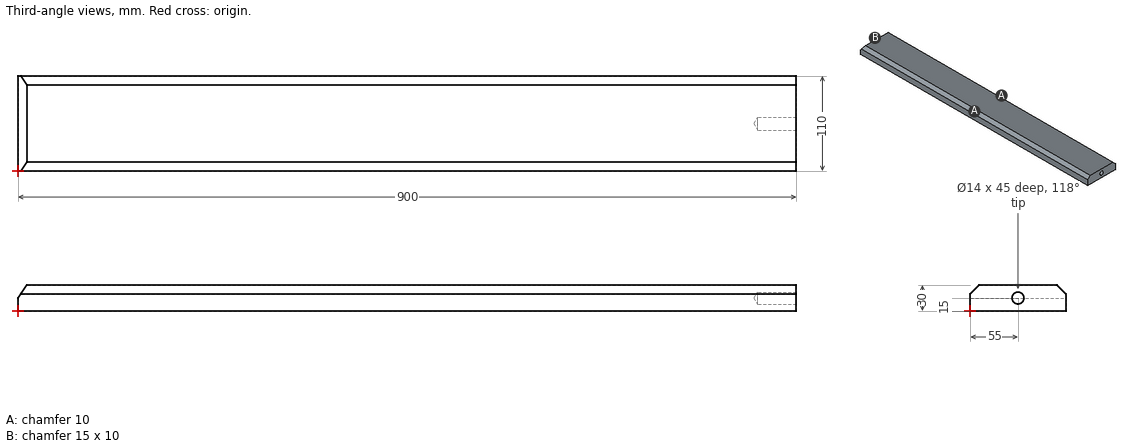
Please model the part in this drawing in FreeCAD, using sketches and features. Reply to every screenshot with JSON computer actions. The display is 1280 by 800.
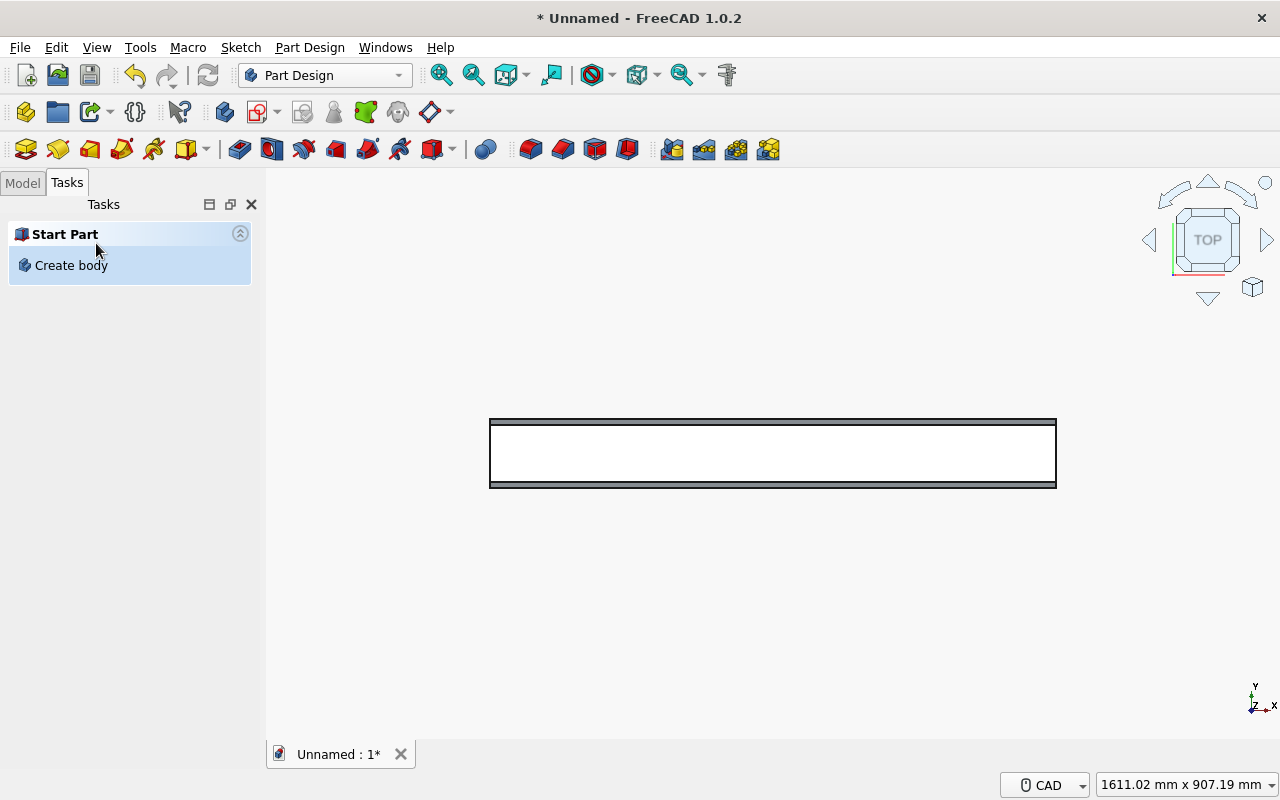
{"action": "left_click", "coordinate": [490, 452]}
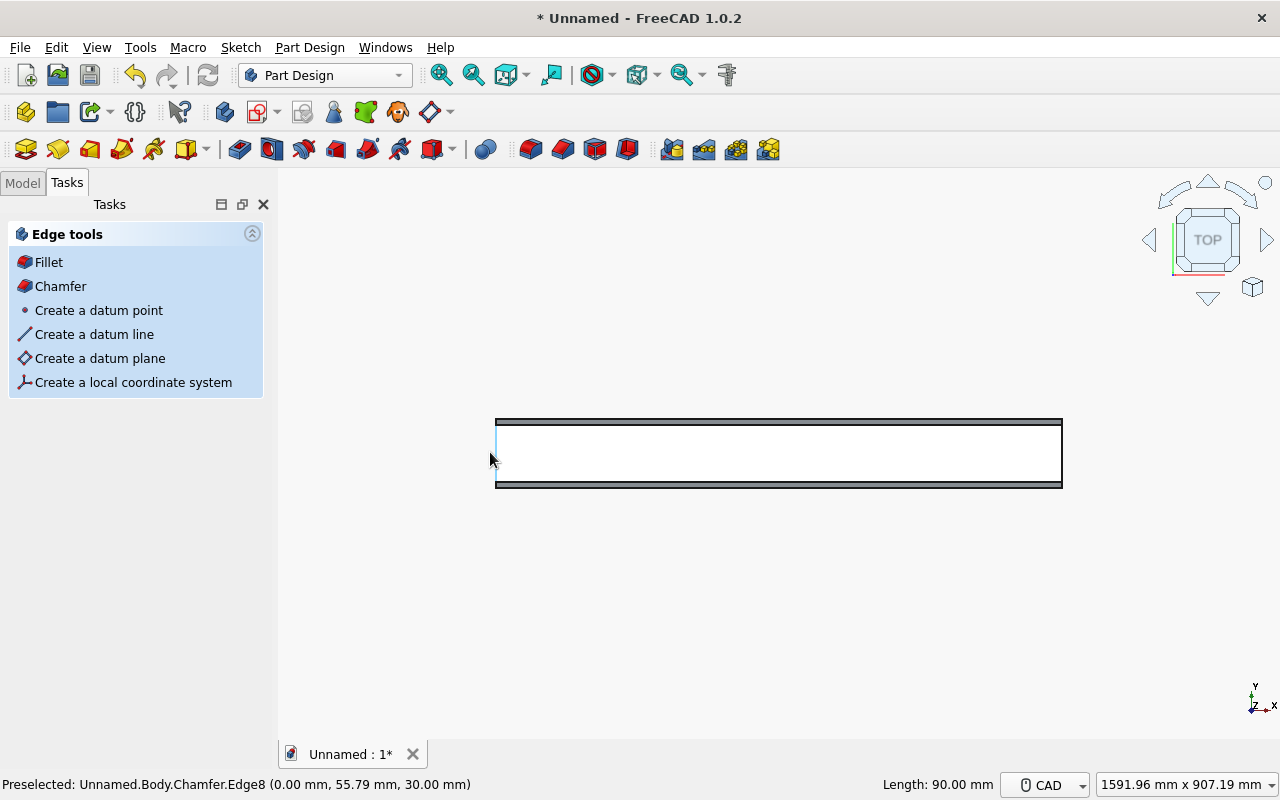
{"action": "left_click", "coordinate": [564, 150]}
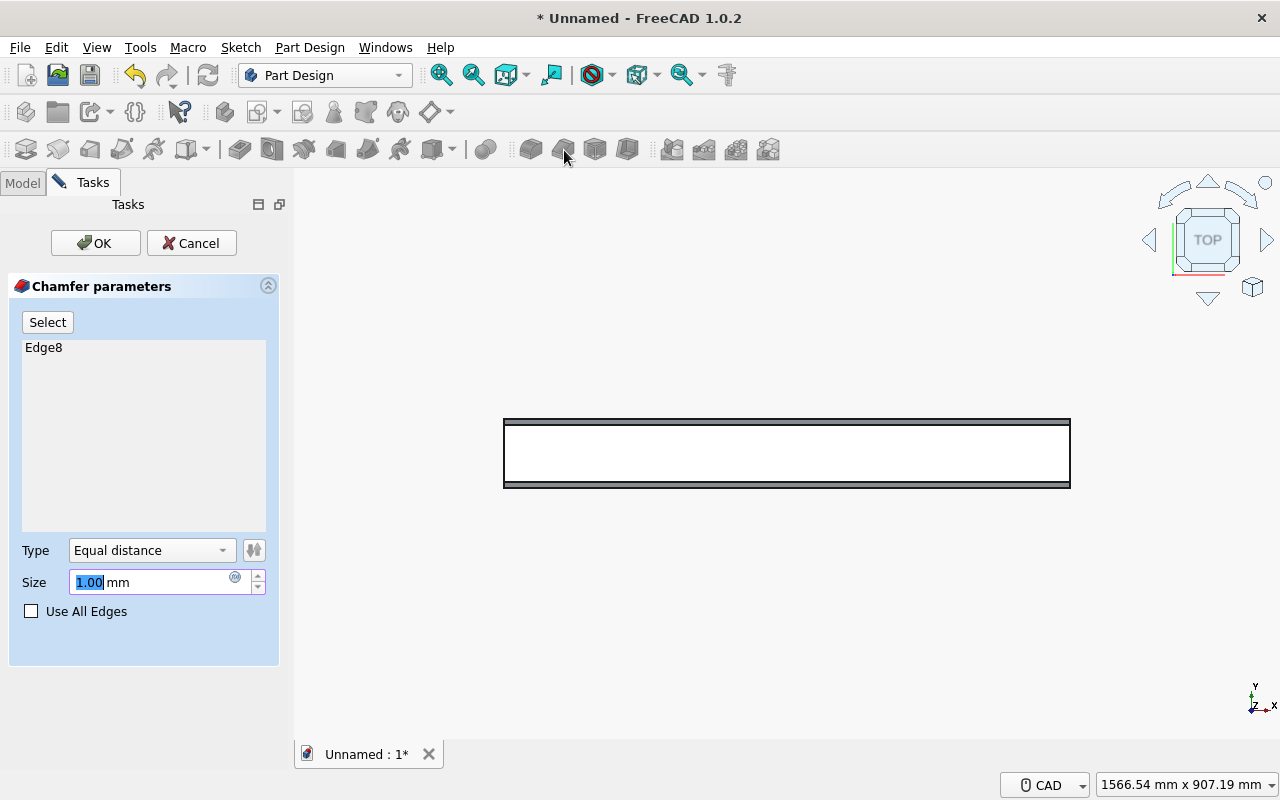
{"action": "type", "text": "15"}
{"action": "key", "text": "Tab"}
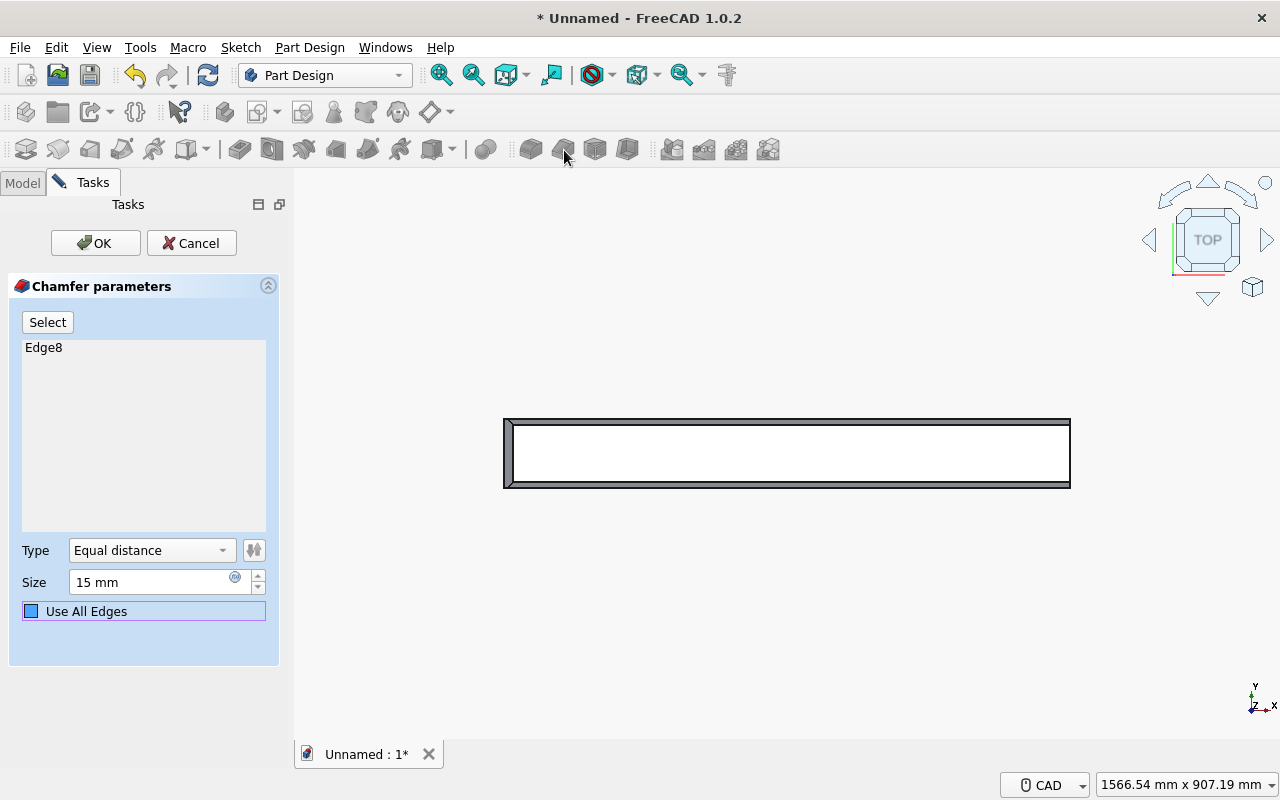
{"action": "left_click", "coordinate": [153, 550]}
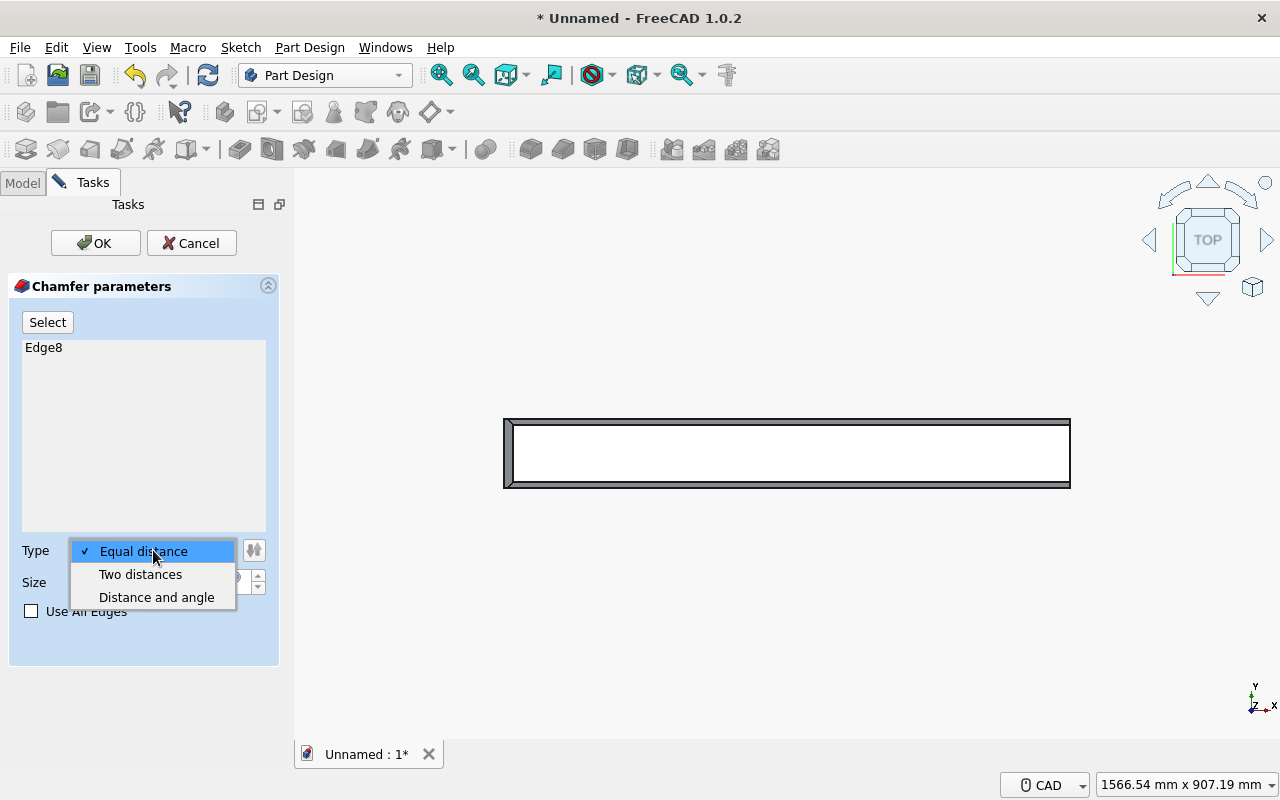
{"action": "left_click", "coordinate": [152, 574]}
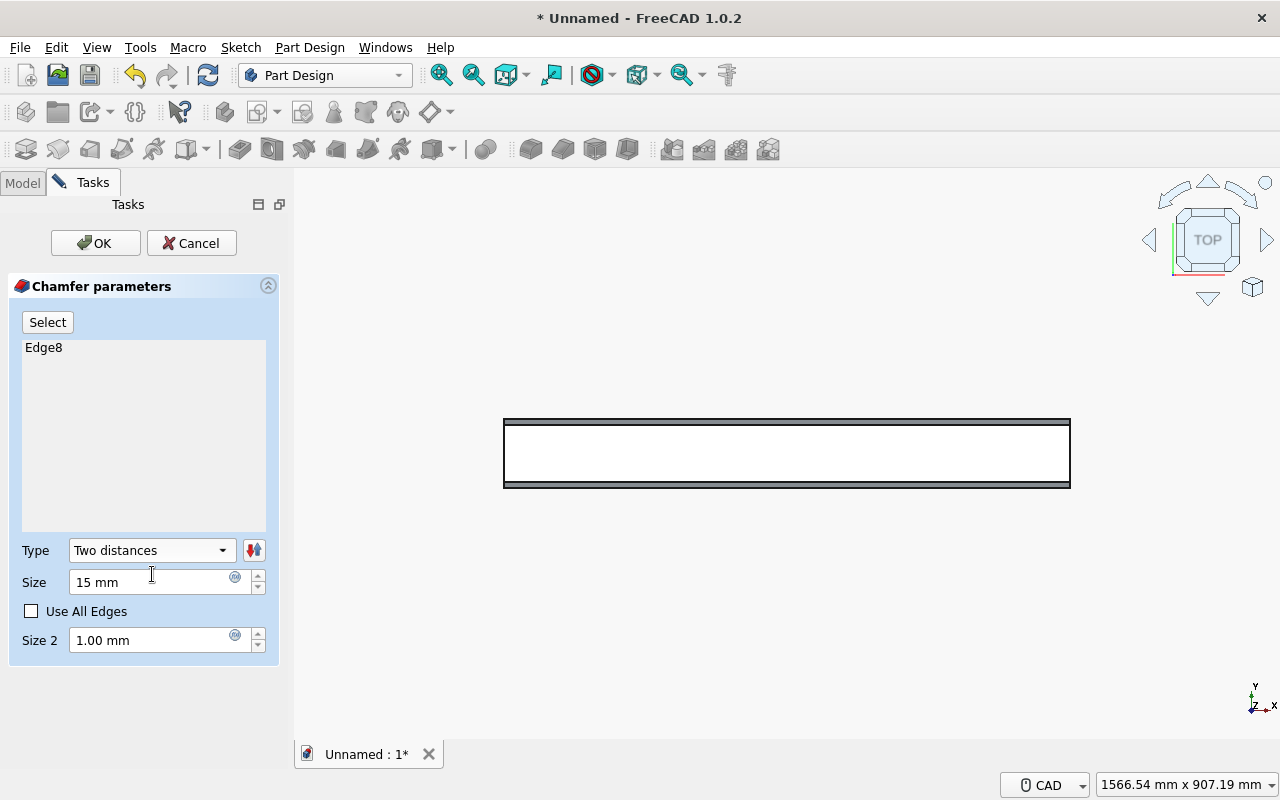
{"action": "triple_click", "coordinate": [160, 640]}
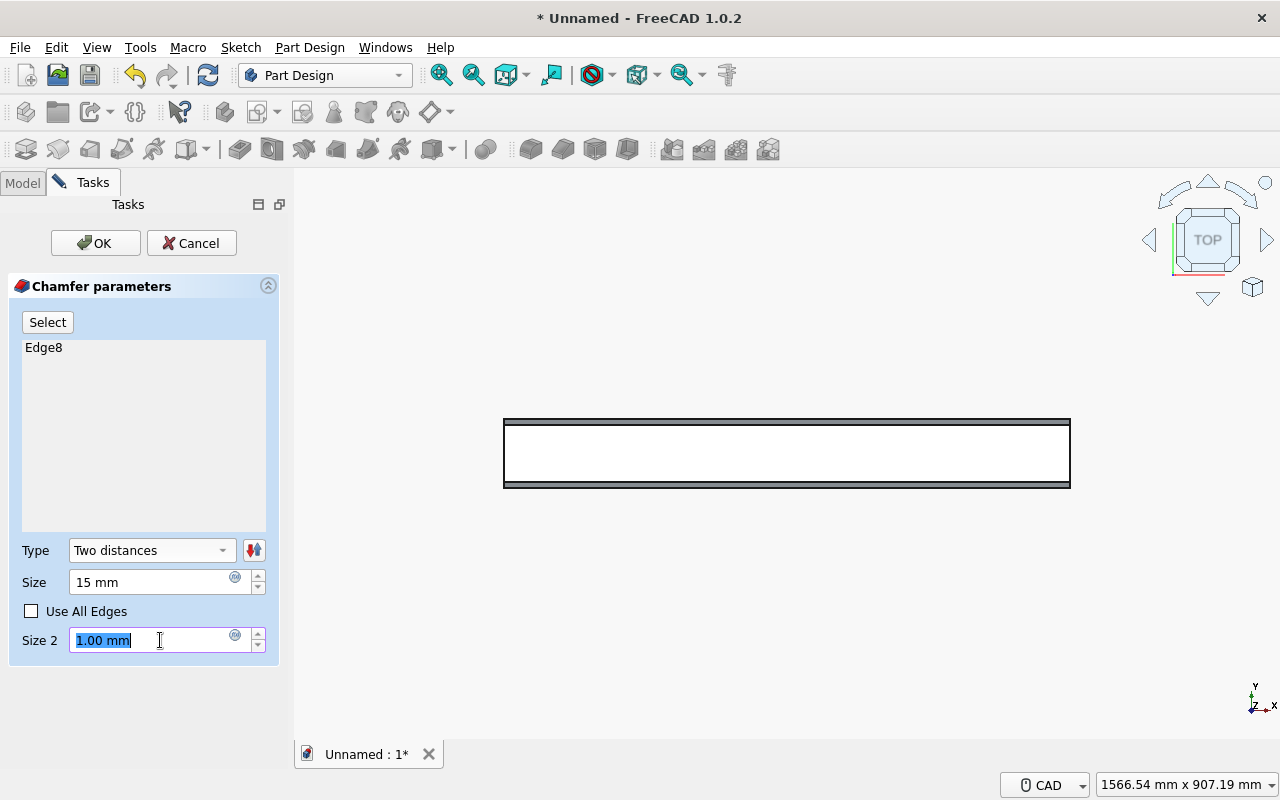
{"action": "type", "text": "10"}
{"action": "key", "text": "Tab"}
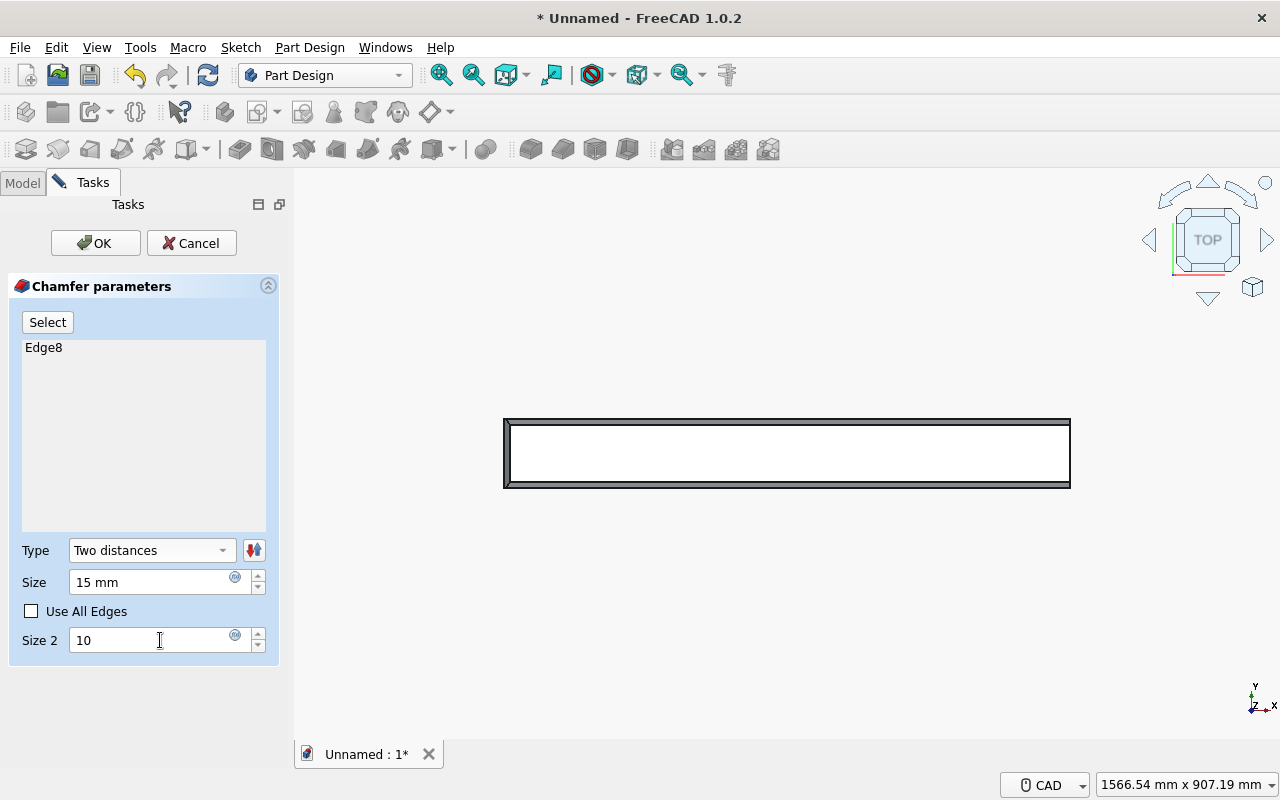
{"action": "left_click", "coordinate": [96, 243]}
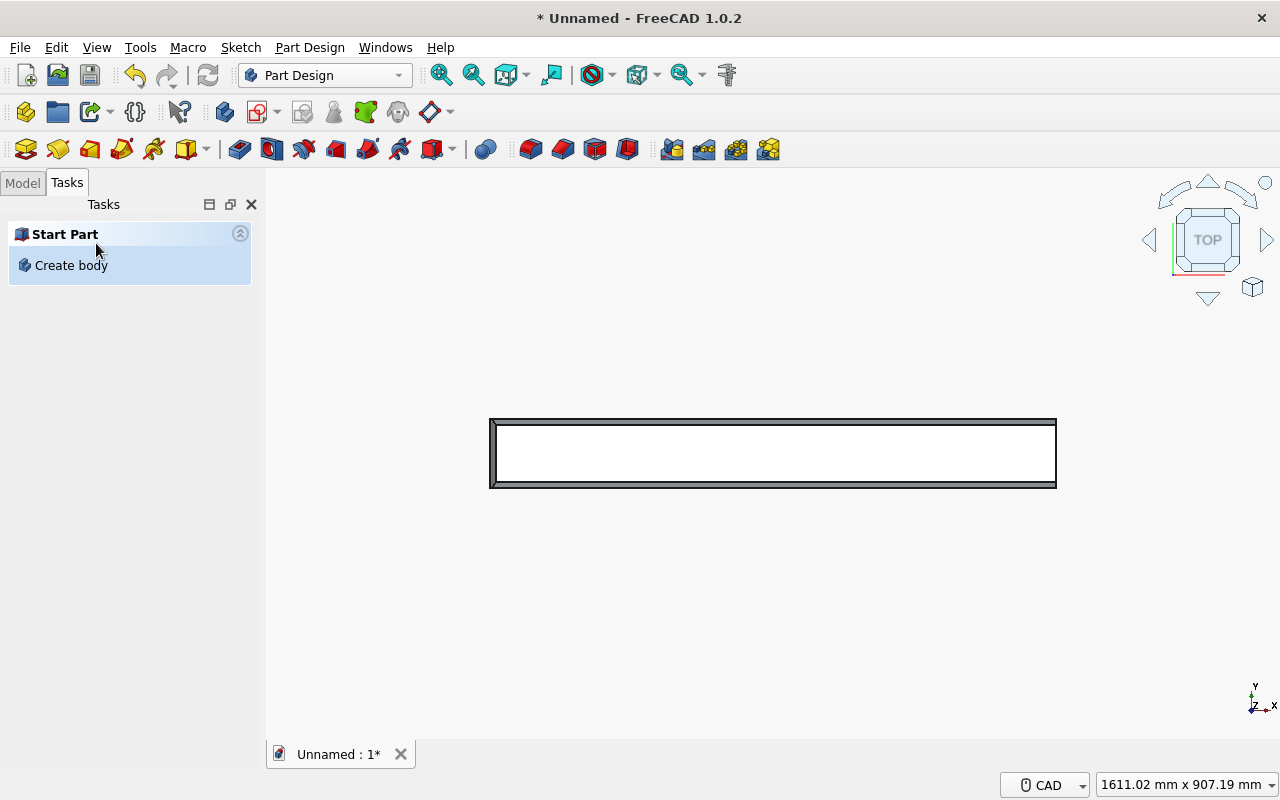
{"action": "key", "text": "0"}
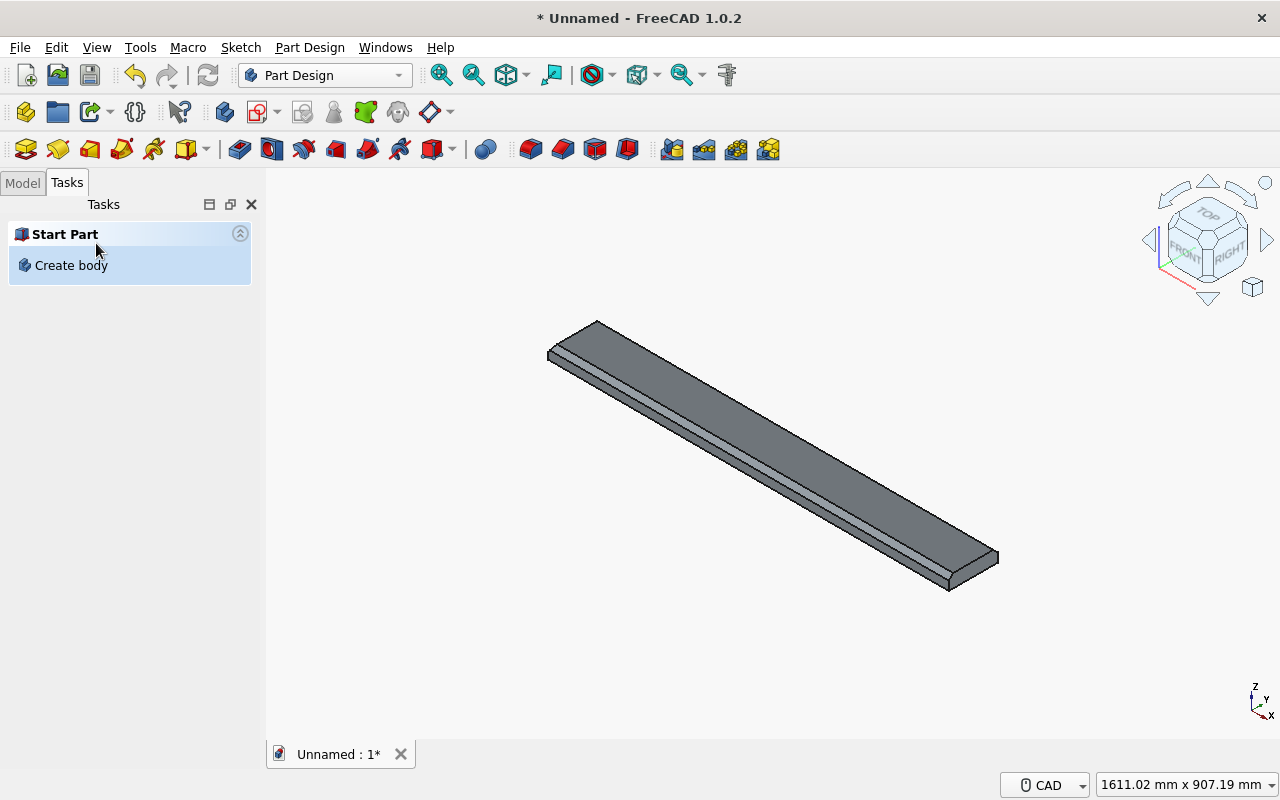
{"action": "key", "text": "3"}